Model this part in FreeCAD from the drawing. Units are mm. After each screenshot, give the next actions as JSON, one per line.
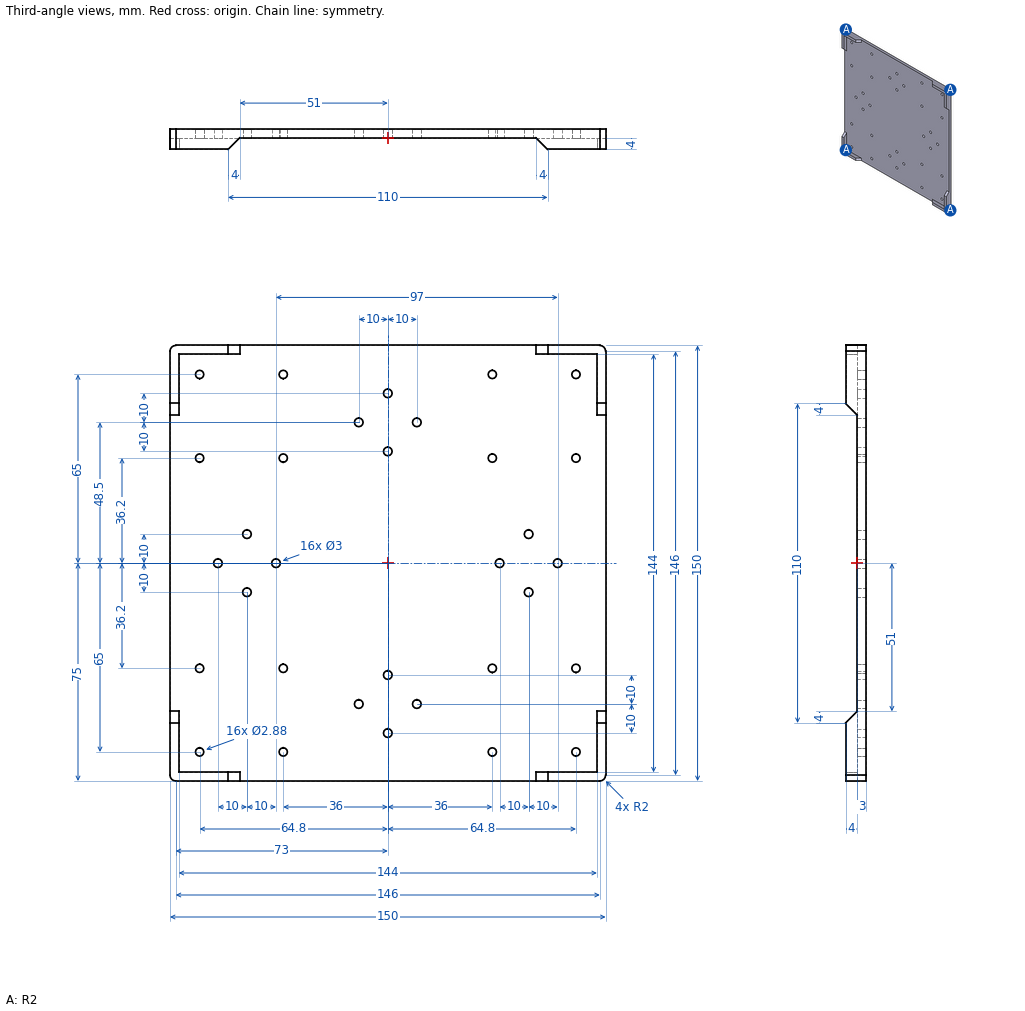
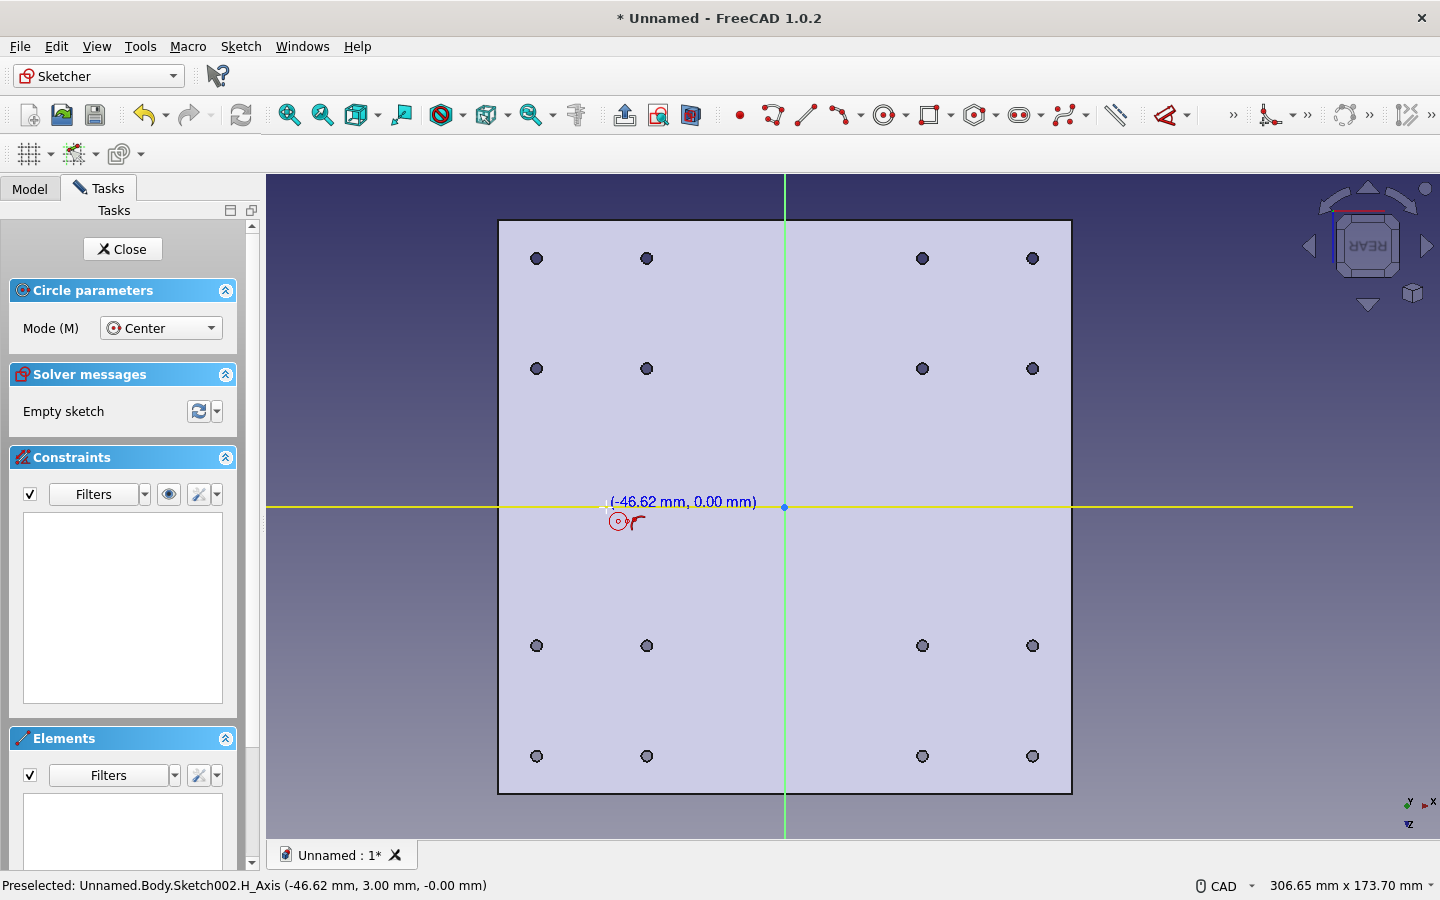
{"action": "left_click", "coordinate": [637, 507]}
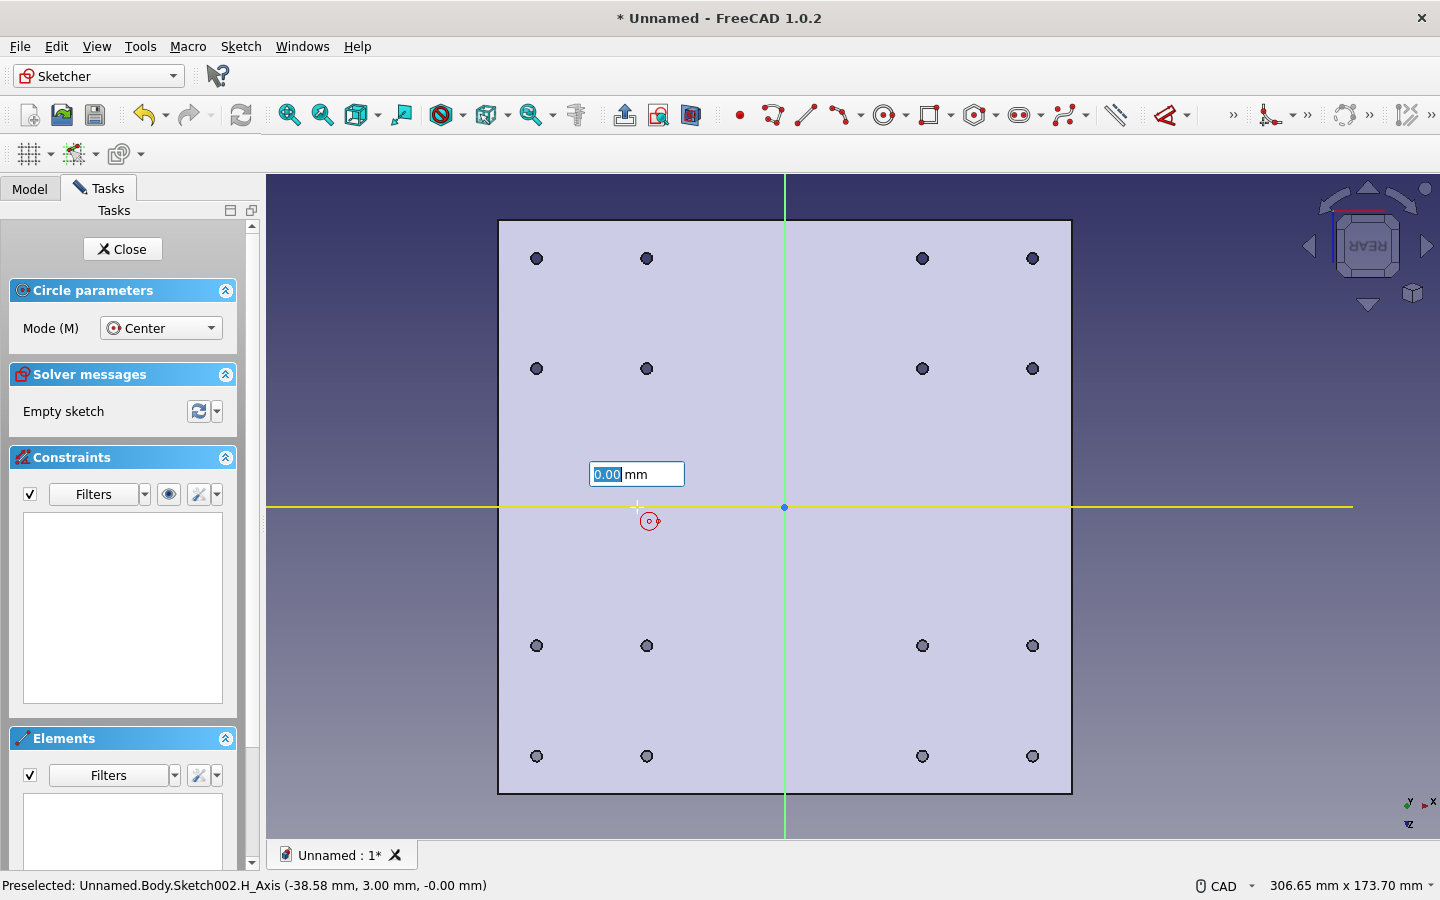
{"action": "scroll", "coordinate": [635, 513], "scroll_direction": "up", "scroll_amount": 6}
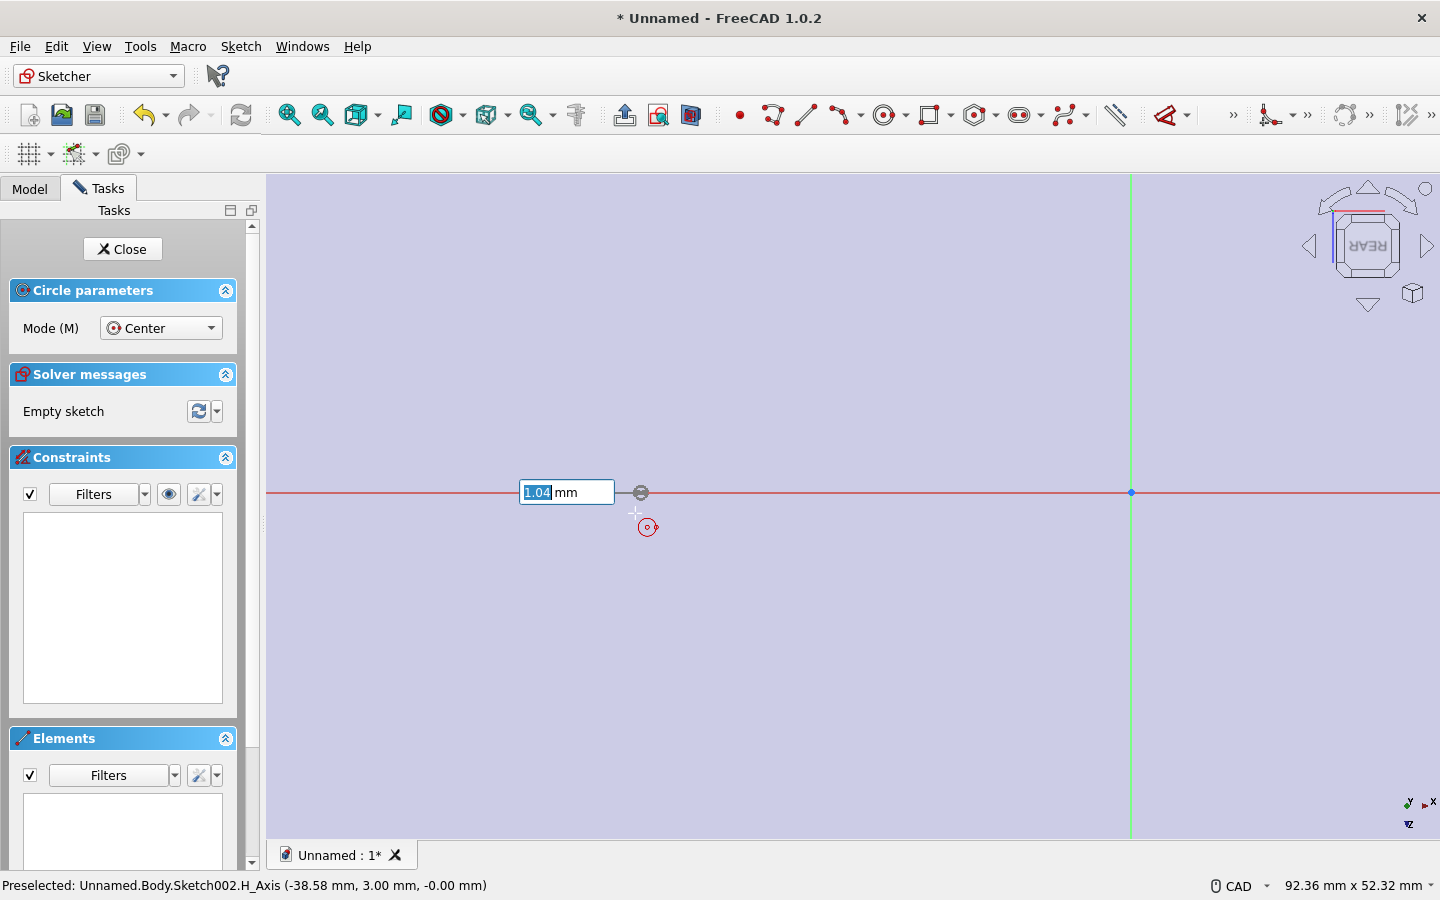
{"action": "left_click", "coordinate": [635, 511]}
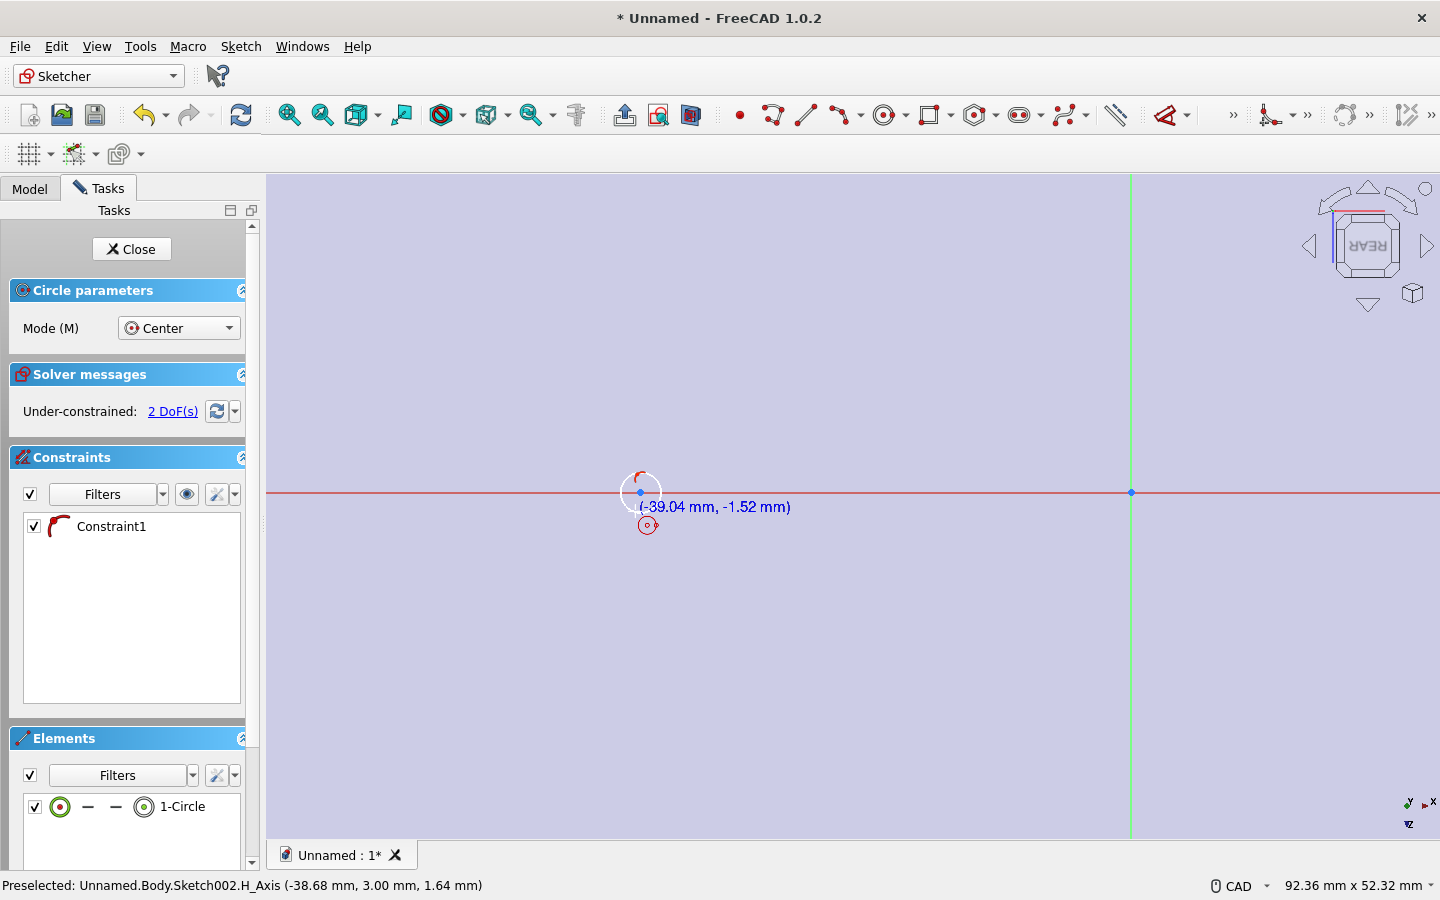
{"action": "scroll", "coordinate": [635, 512], "scroll_direction": "down", "scroll_amount": 6}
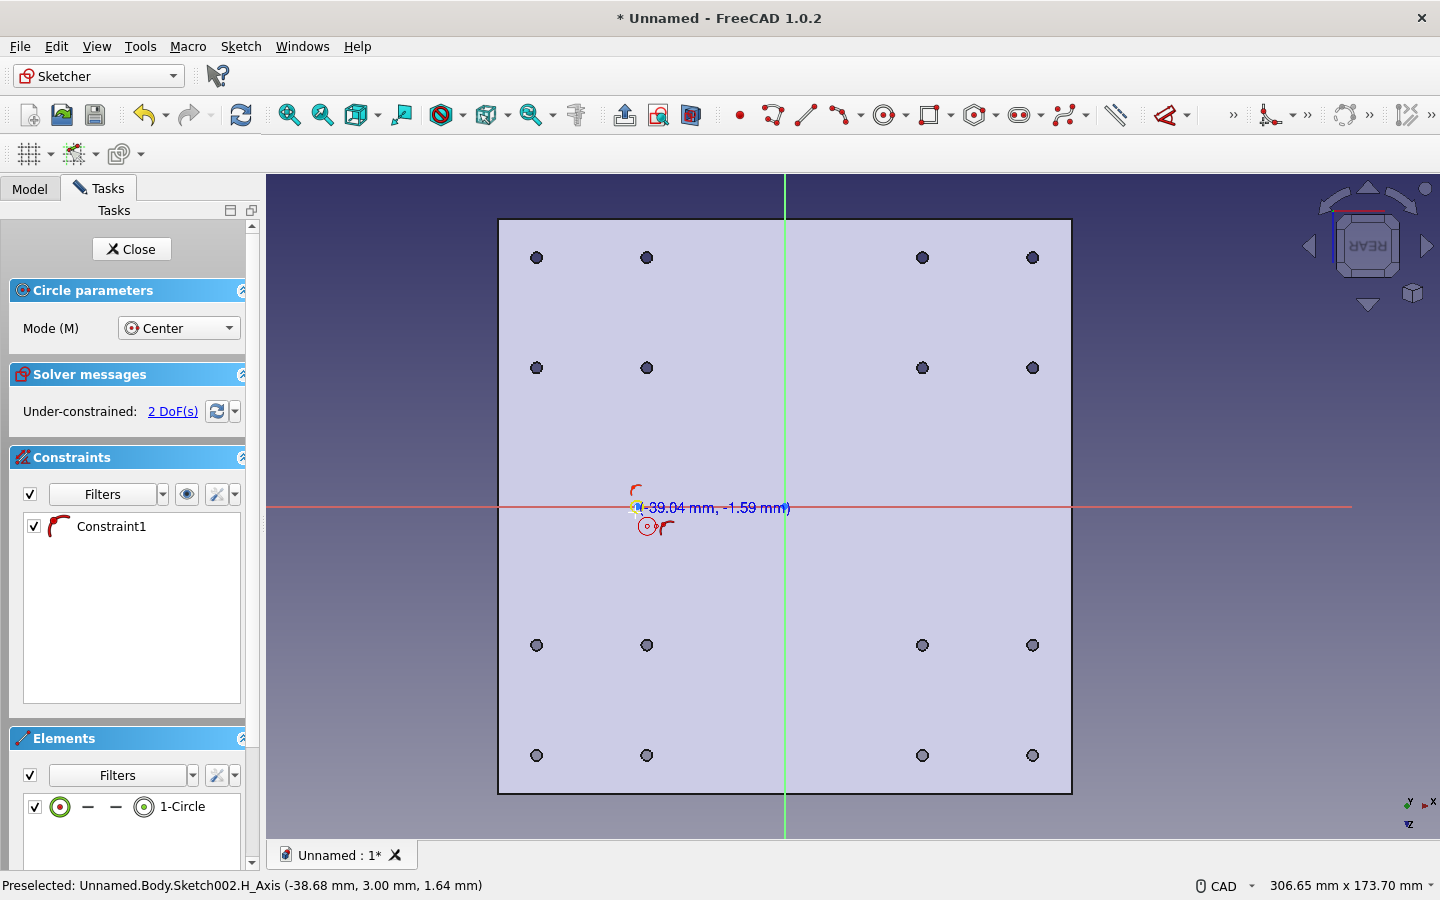
{"action": "left_click", "coordinate": [599, 468]}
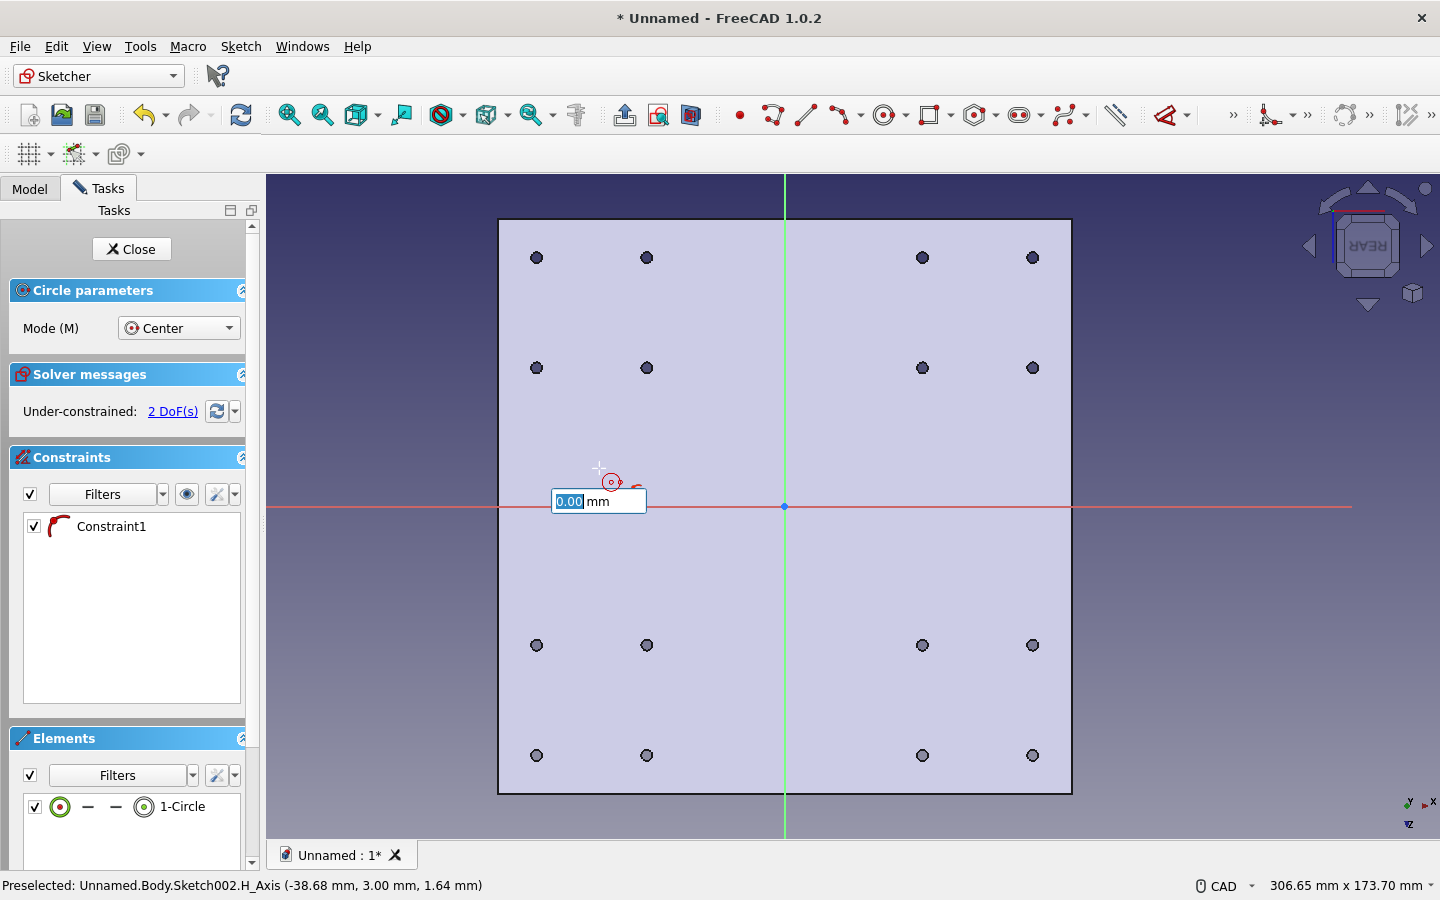
{"action": "scroll", "coordinate": [603, 464], "scroll_direction": "up", "scroll_amount": 6}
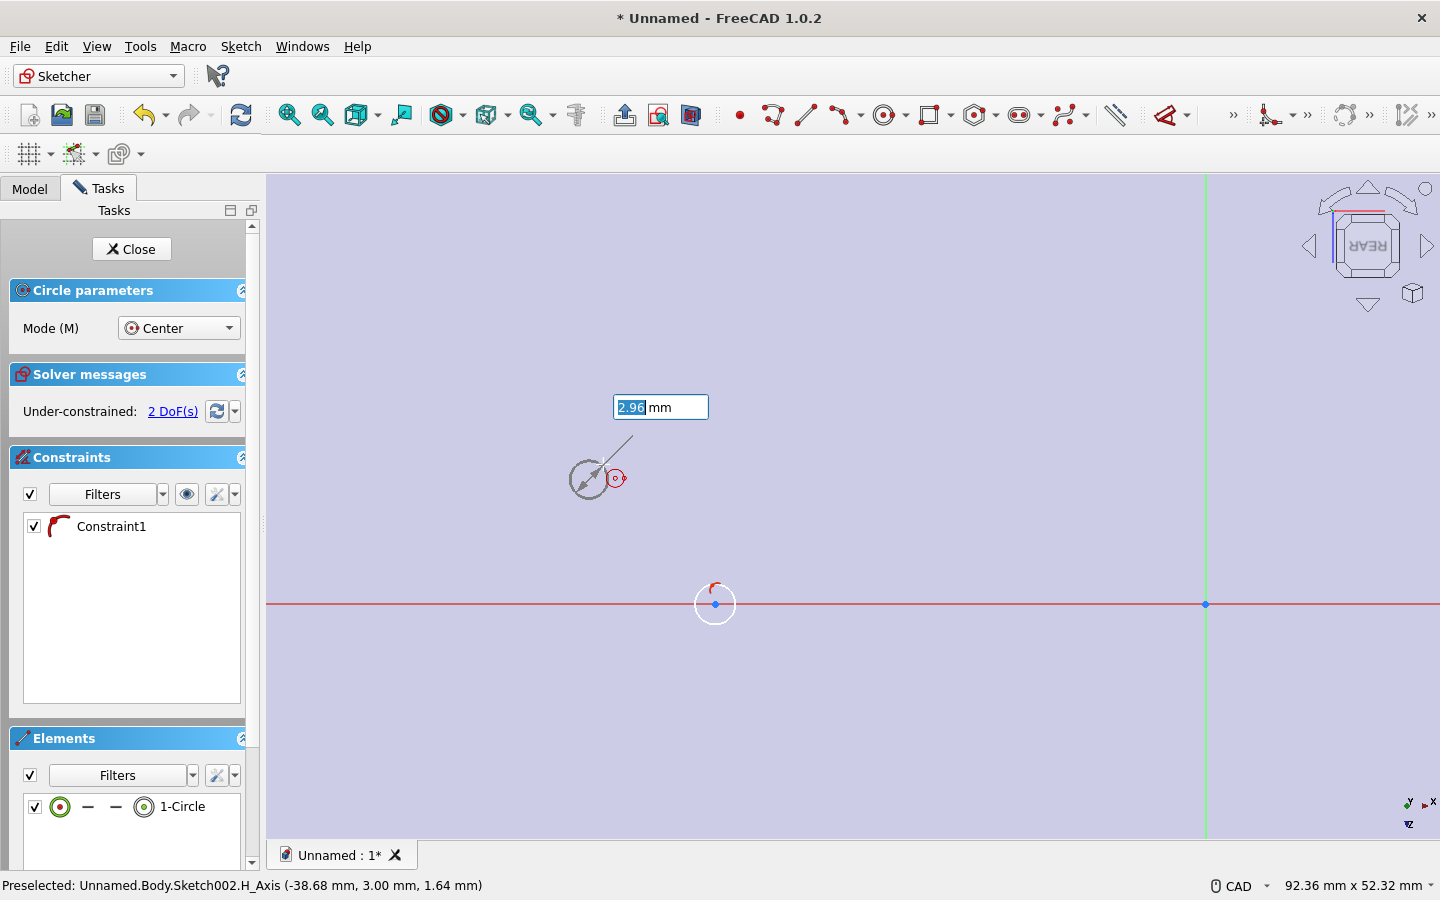
{"action": "left_click", "coordinate": [603, 464]}